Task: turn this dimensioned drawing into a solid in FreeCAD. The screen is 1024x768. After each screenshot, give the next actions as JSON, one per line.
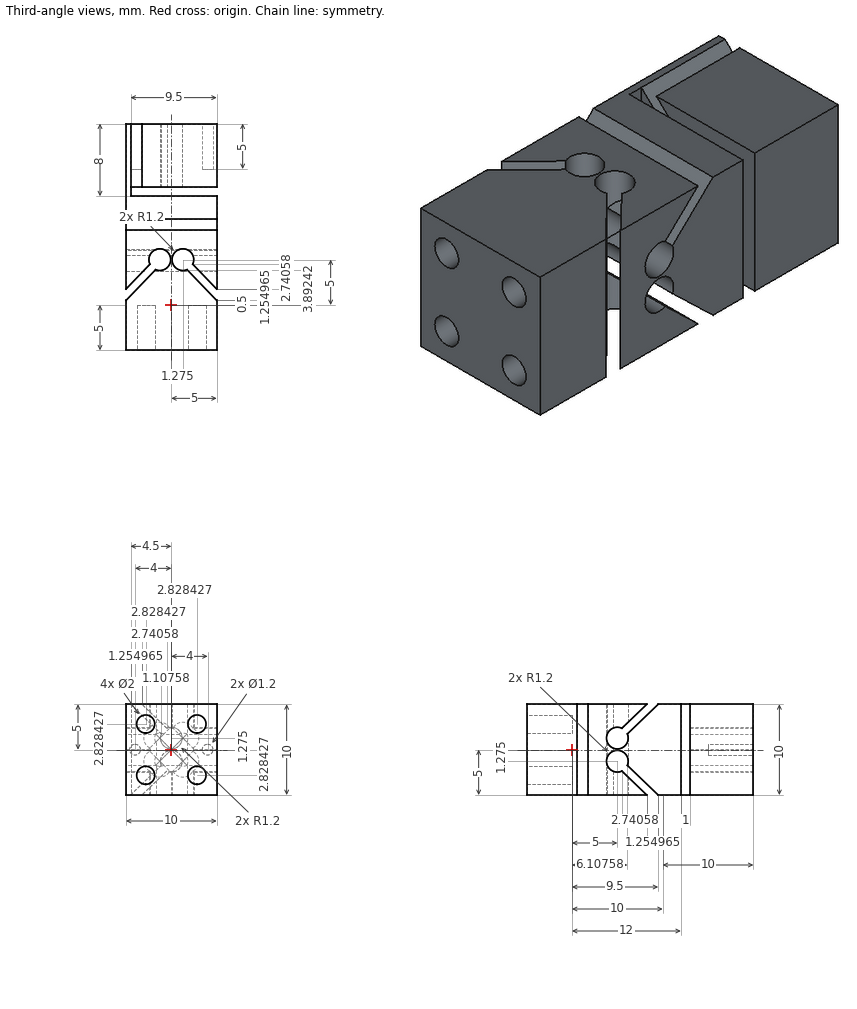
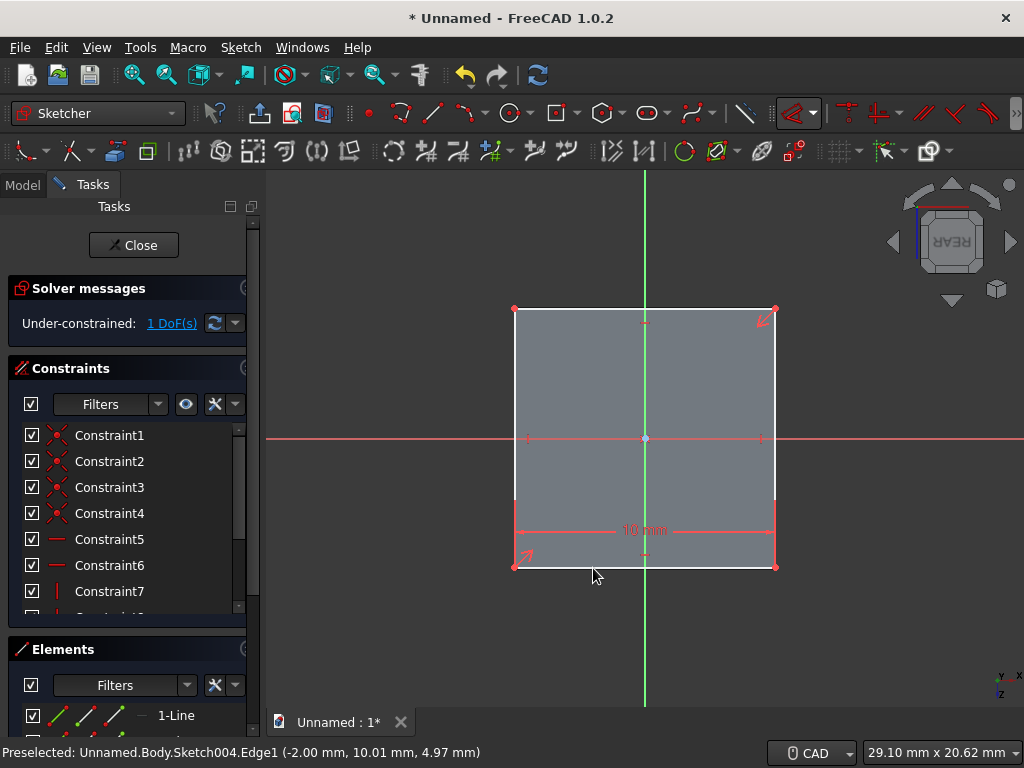
{"action": "left_click", "coordinate": [775, 490]}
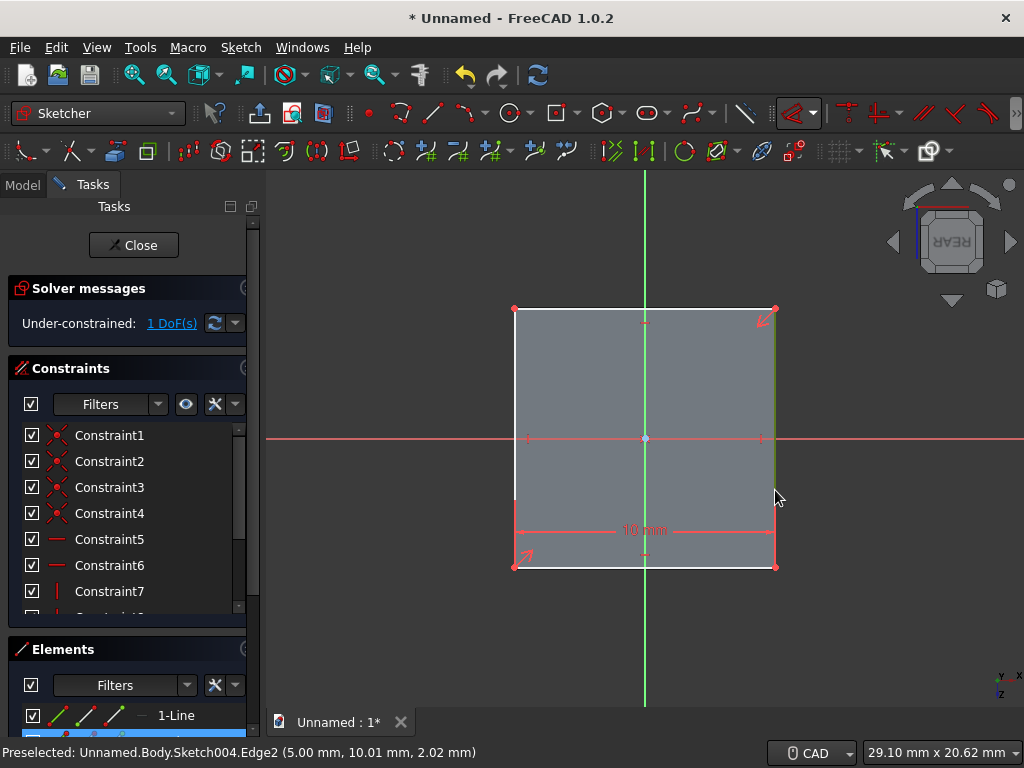
{"action": "left_click", "coordinate": [816, 114]}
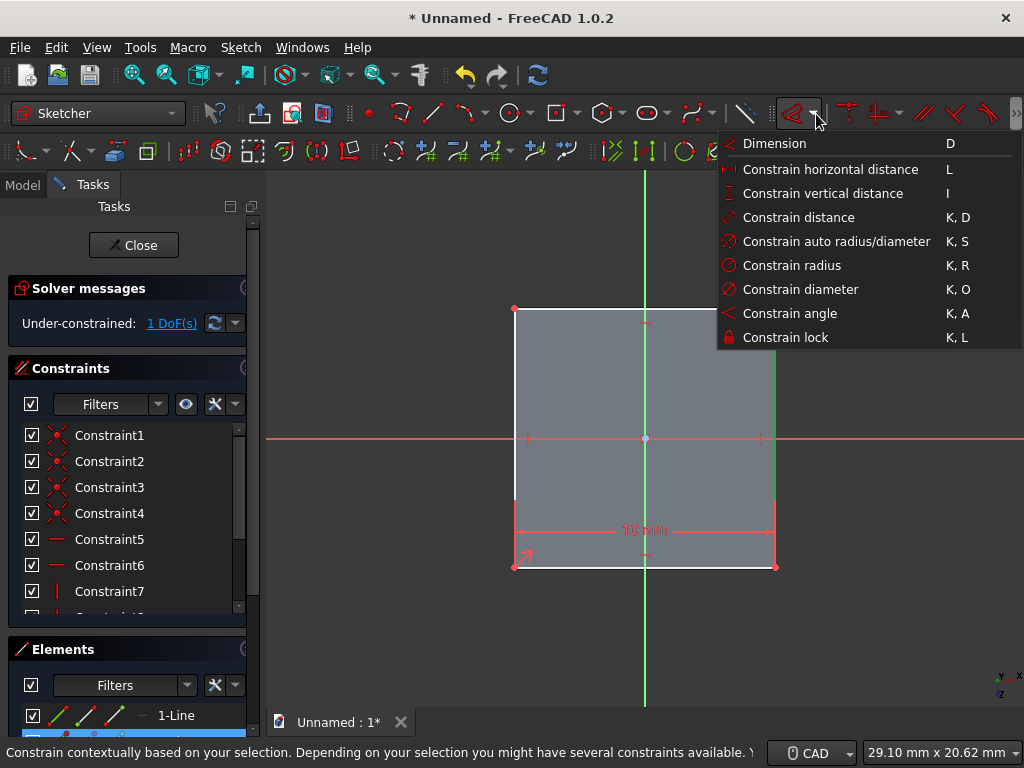
{"action": "left_click", "coordinate": [870, 193]}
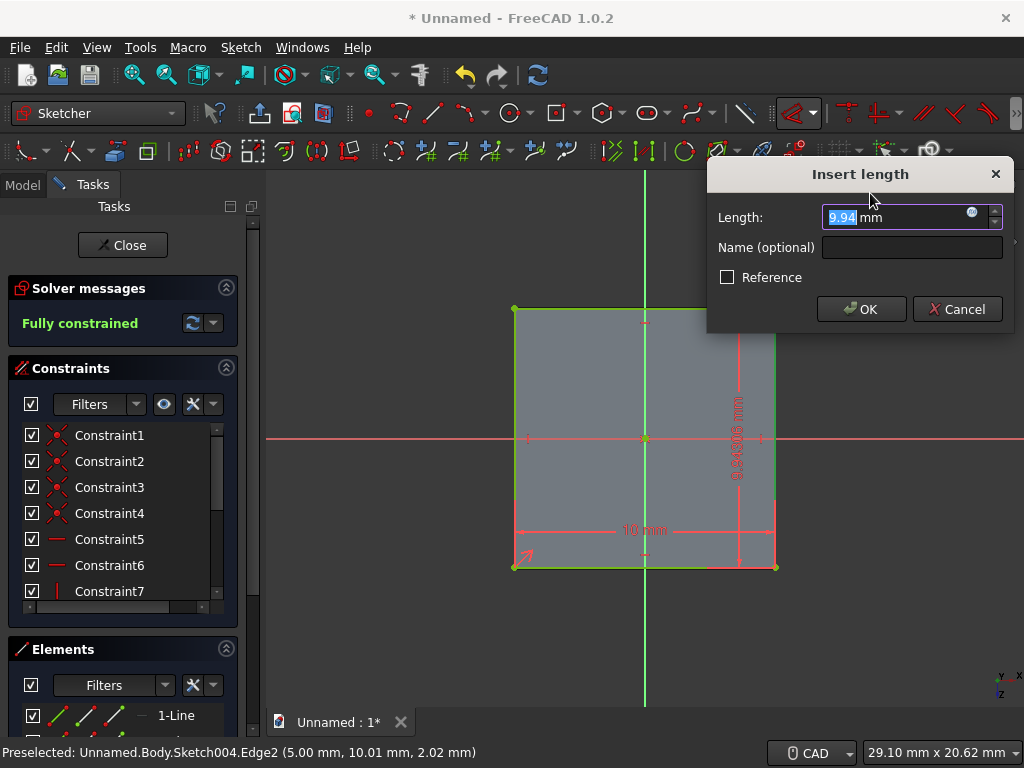
{"action": "type", "text": "10"}
{"action": "key", "text": "Return"}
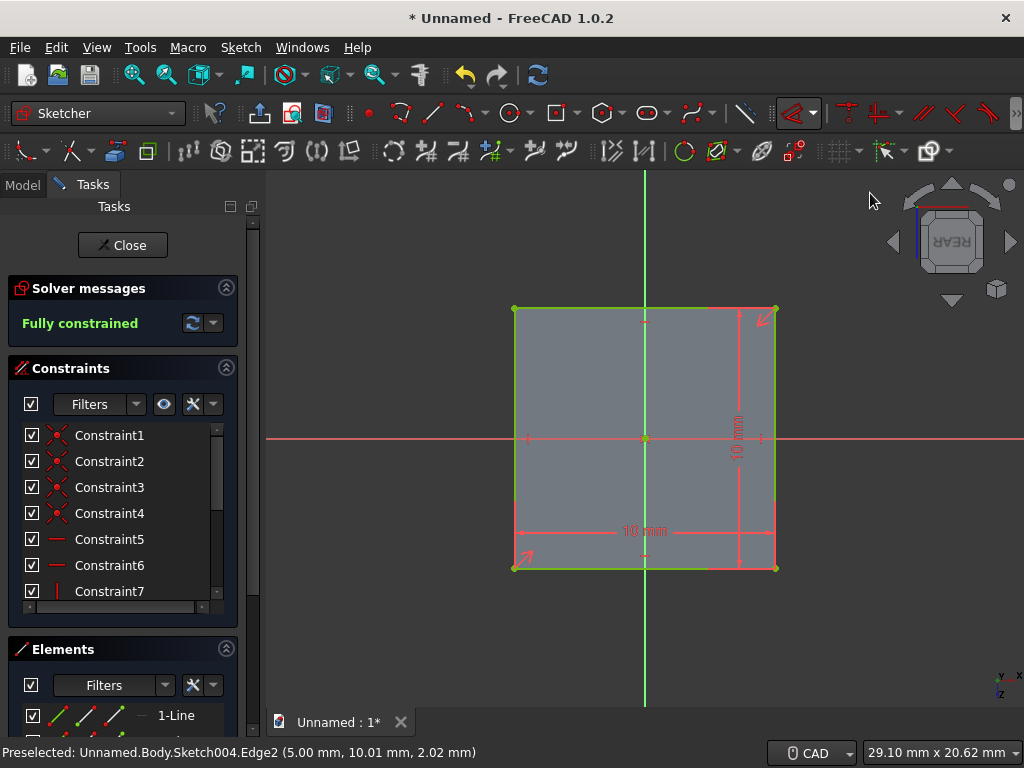
{"action": "left_click", "coordinate": [123, 245]}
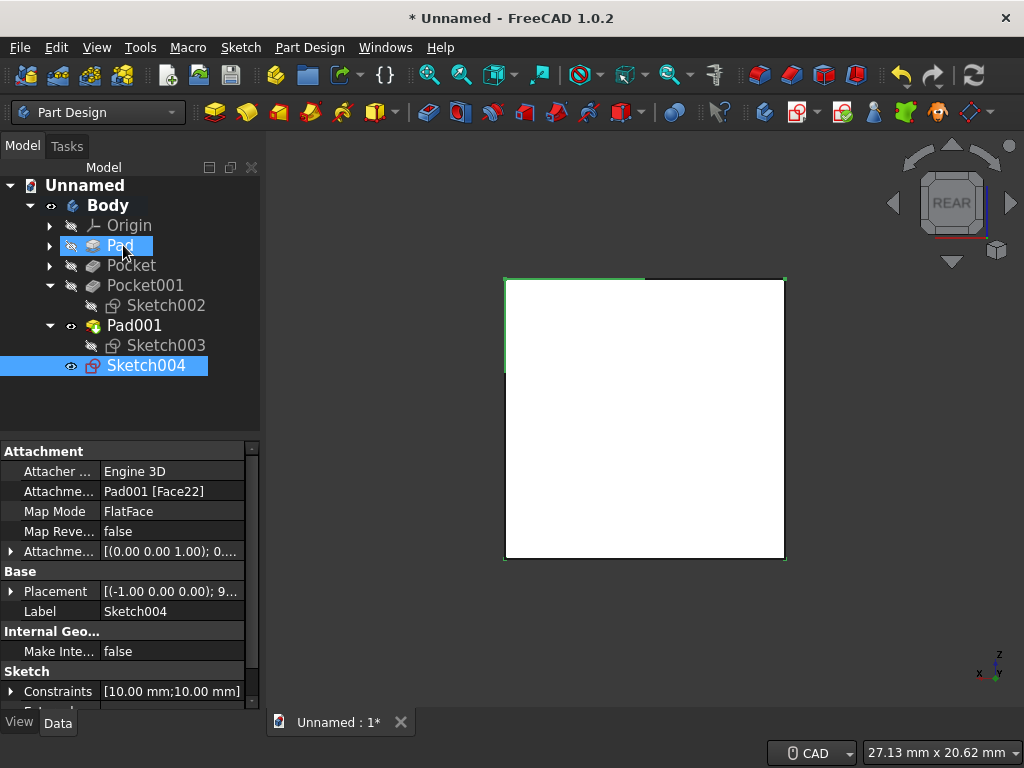
{"action": "left_click", "coordinate": [216, 112]}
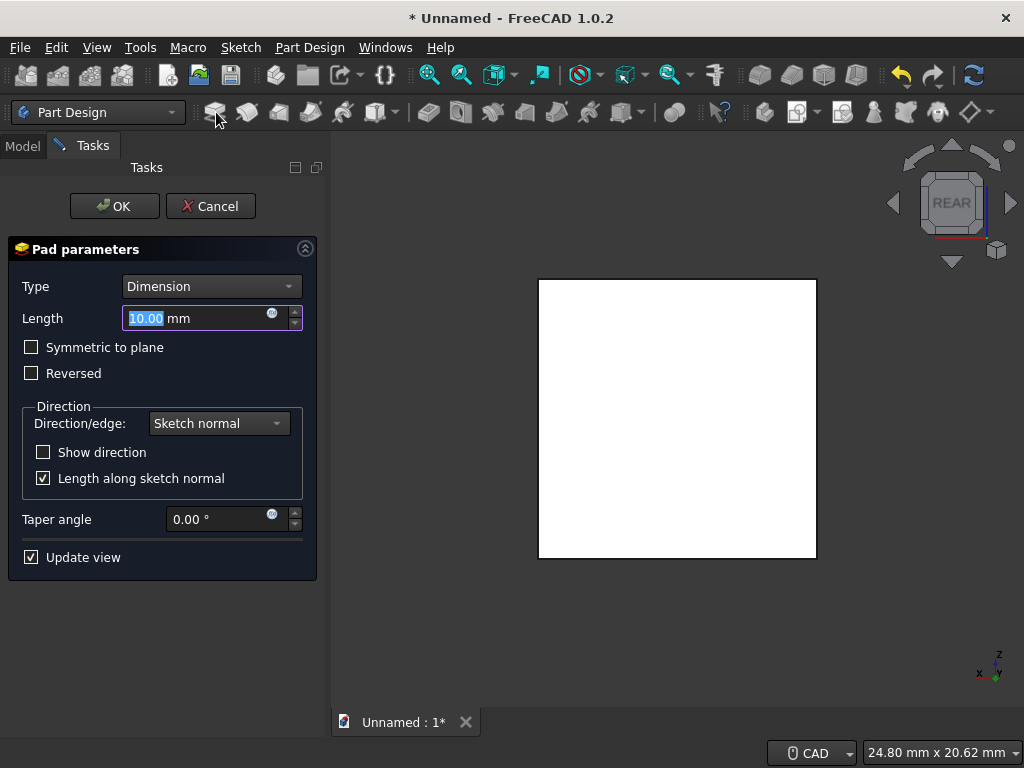
{"action": "type", "text": "10"}
{"action": "key", "text": "Tab"}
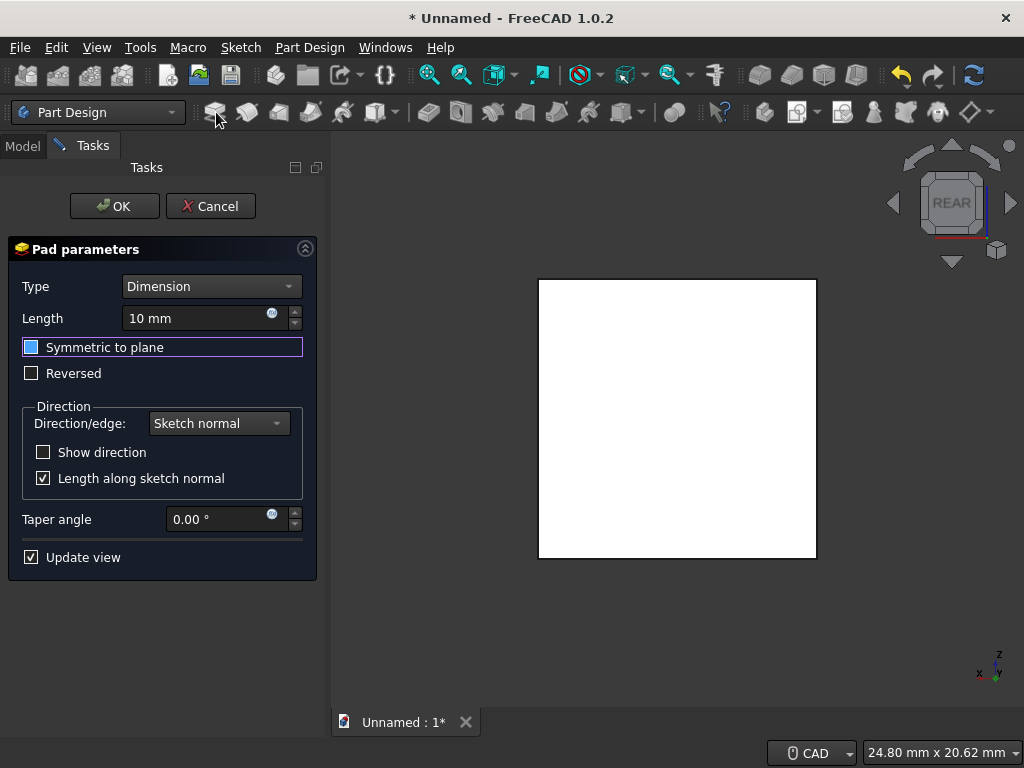
{"action": "left_click", "coordinate": [115, 206]}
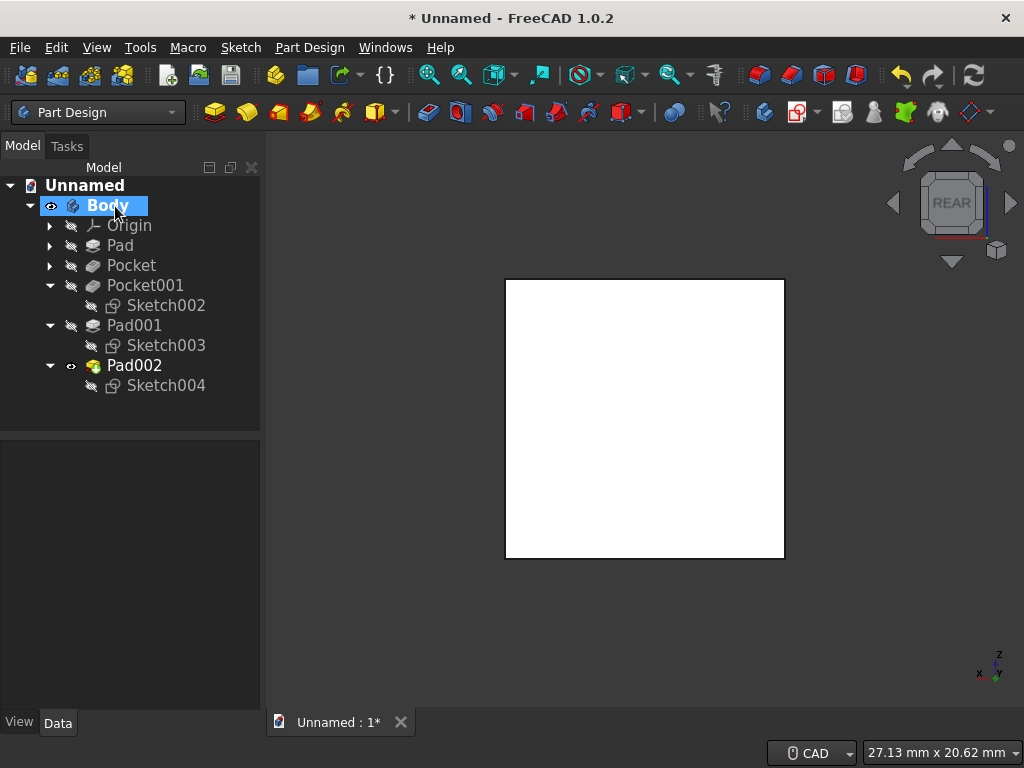
{"action": "left_click", "coordinate": [645, 418]}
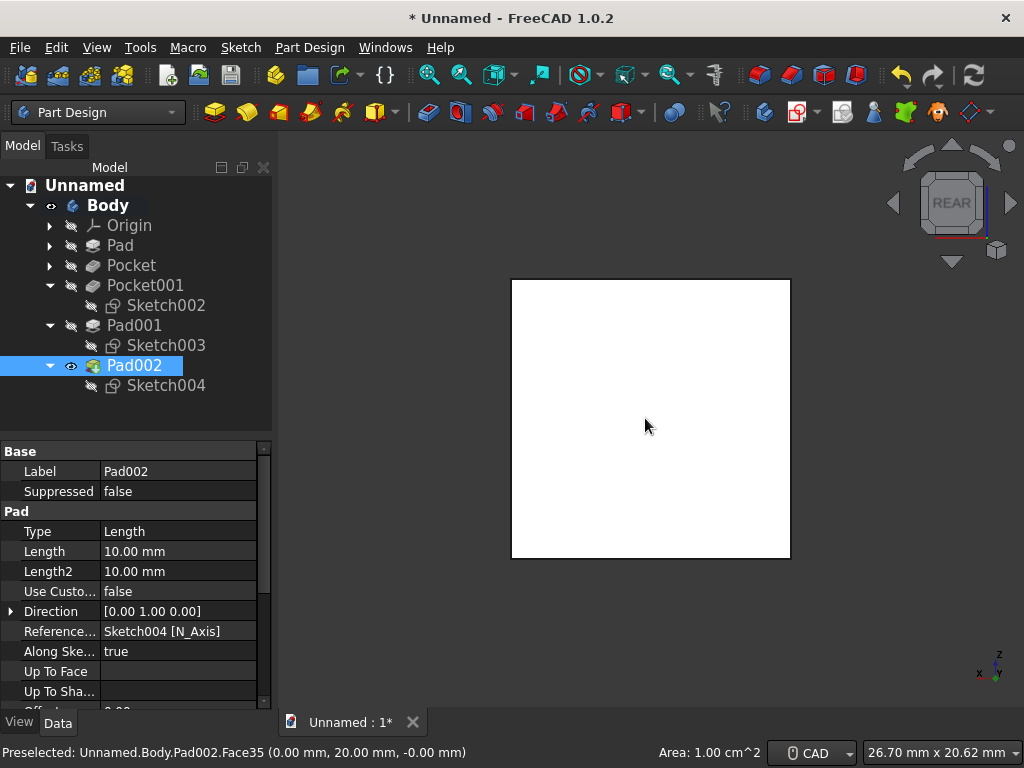
{"action": "left_click", "coordinate": [798, 112]}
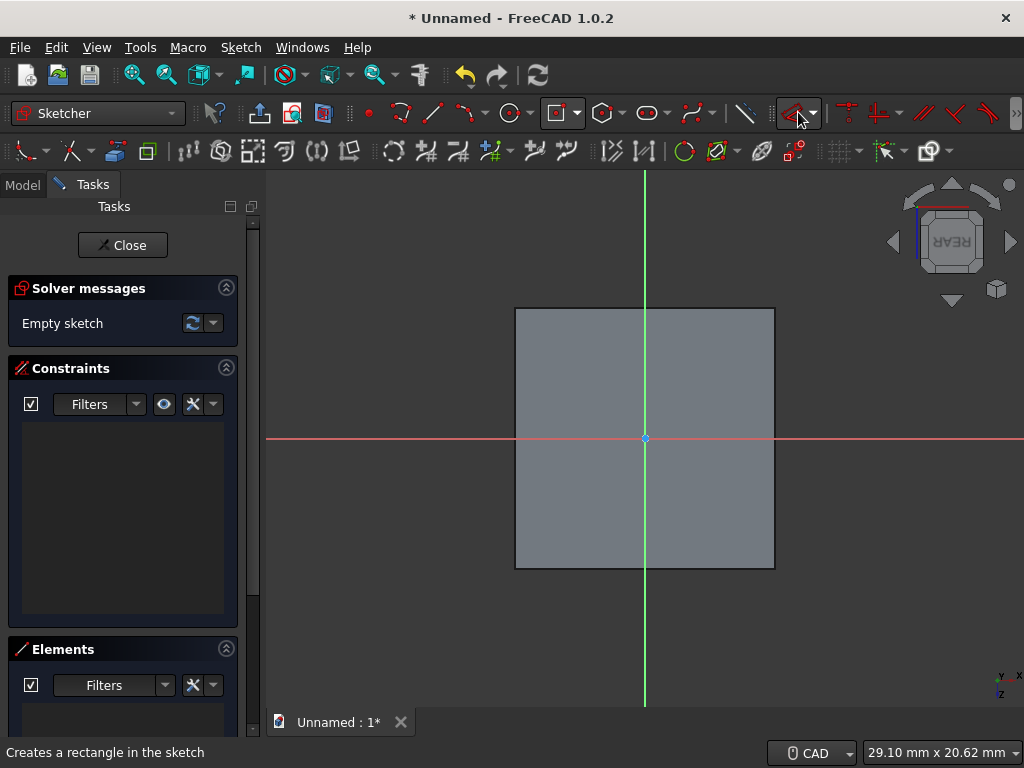
{"action": "left_click", "coordinate": [402, 114]}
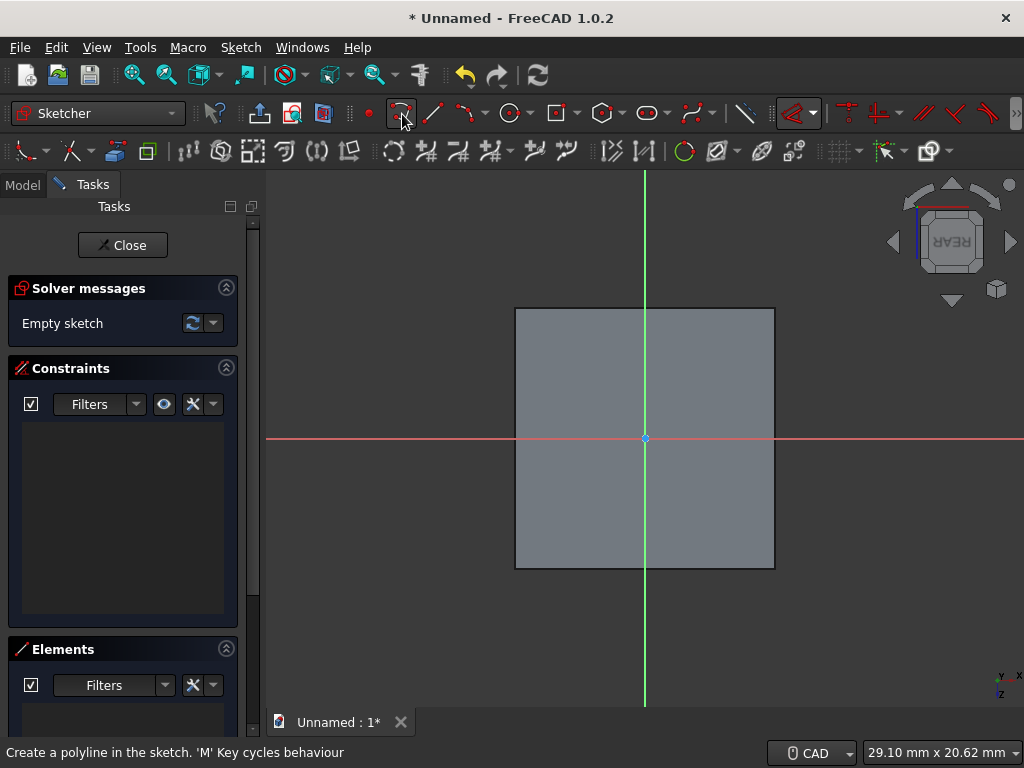
{"action": "left_click", "coordinate": [616, 484]}
{"action": "left_click", "coordinate": [528, 569]}
{"action": "left_click", "coordinate": [560, 569]}
{"action": "left_click", "coordinate": [632, 500]}
{"action": "right_click", "coordinate": [632, 500]}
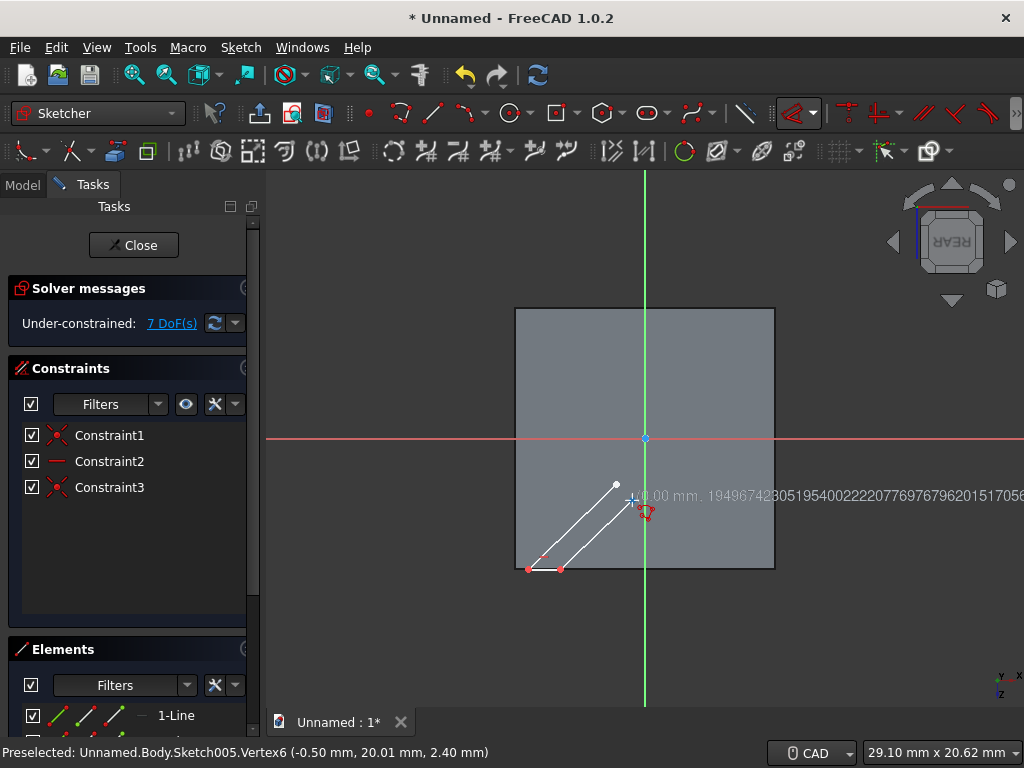
{"action": "left_click", "coordinate": [466, 114]}